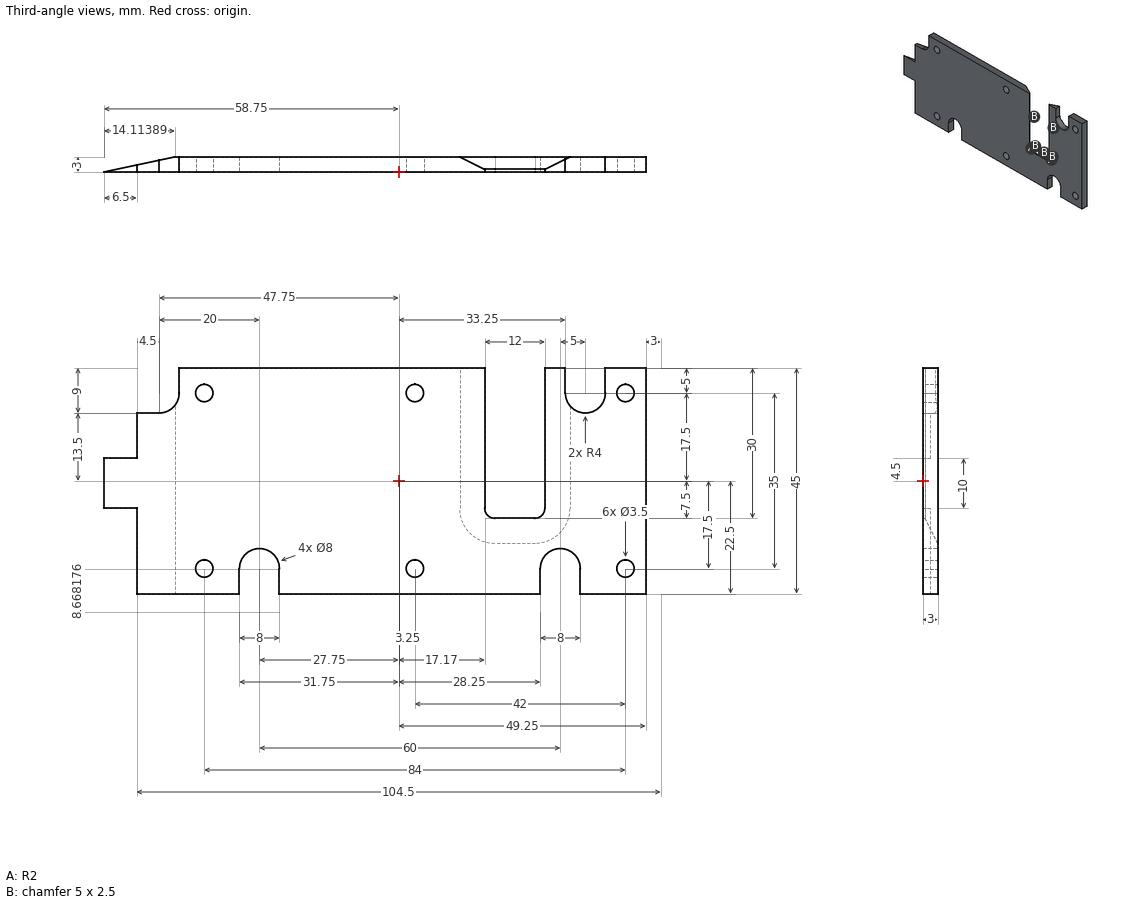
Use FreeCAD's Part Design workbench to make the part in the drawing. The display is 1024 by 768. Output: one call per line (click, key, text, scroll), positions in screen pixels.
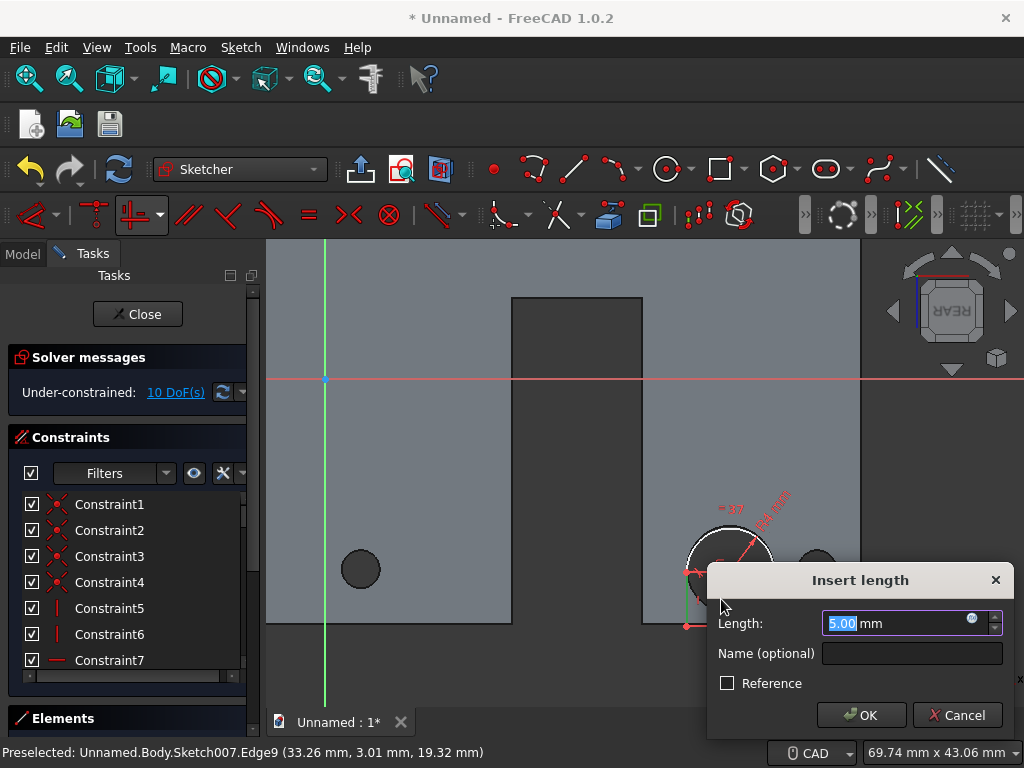
text(5)
key(Return)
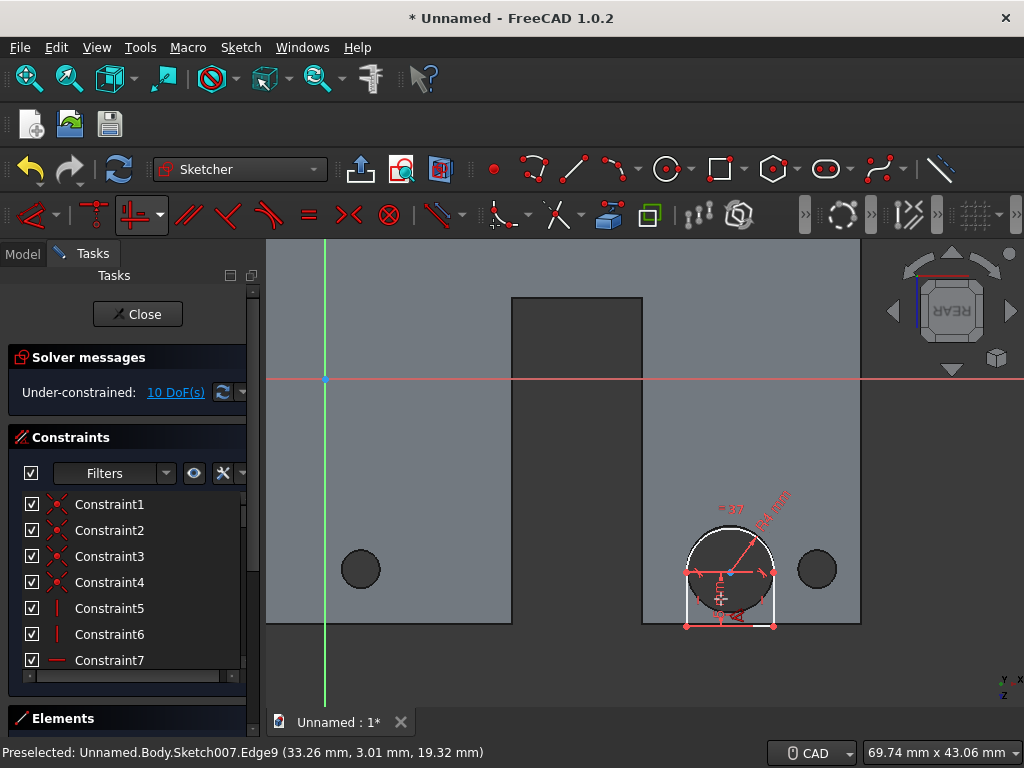
scroll(757, 539, down, 5)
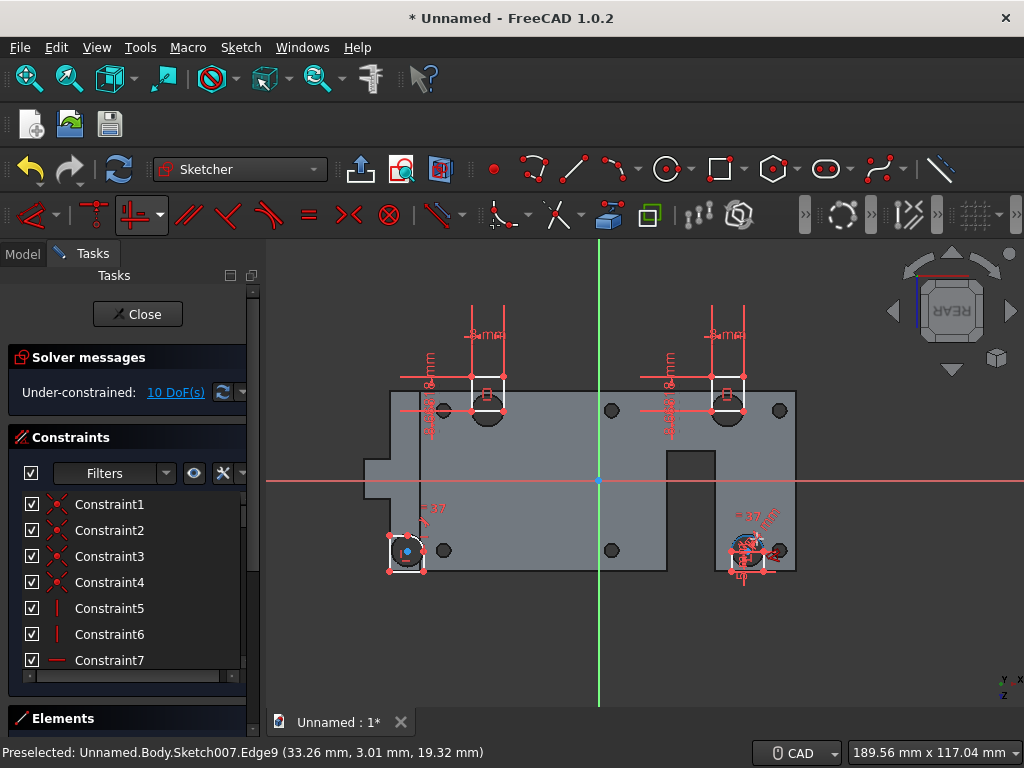
scroll(390, 547, up, 2)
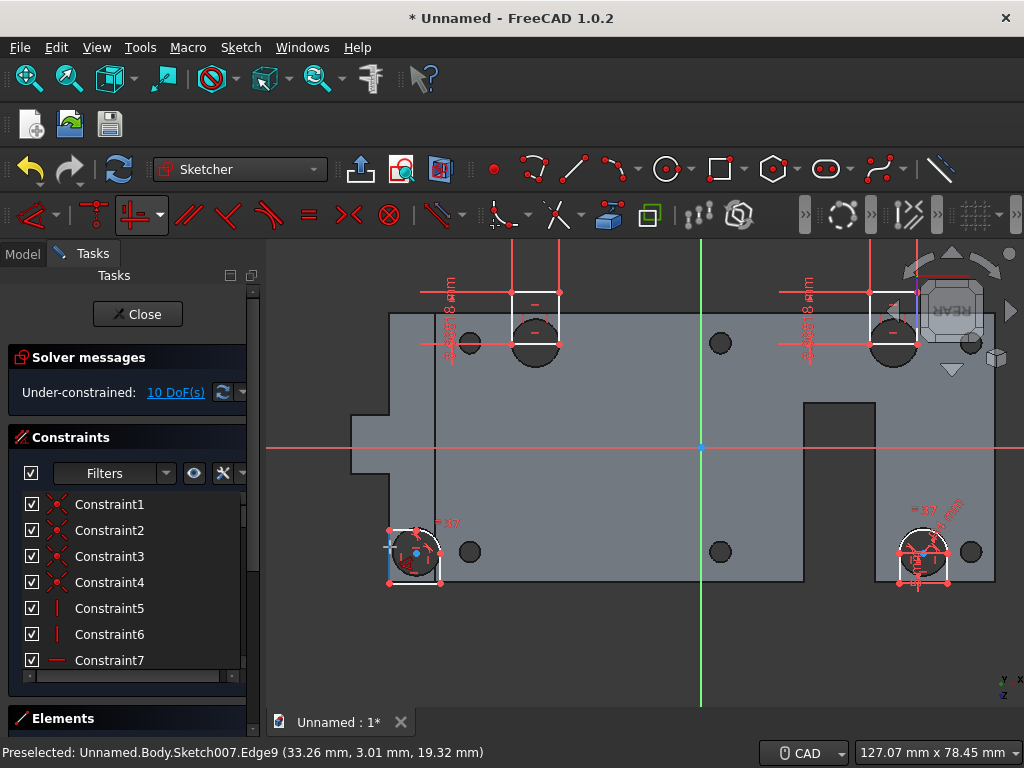
click(389, 546)
click(355, 557)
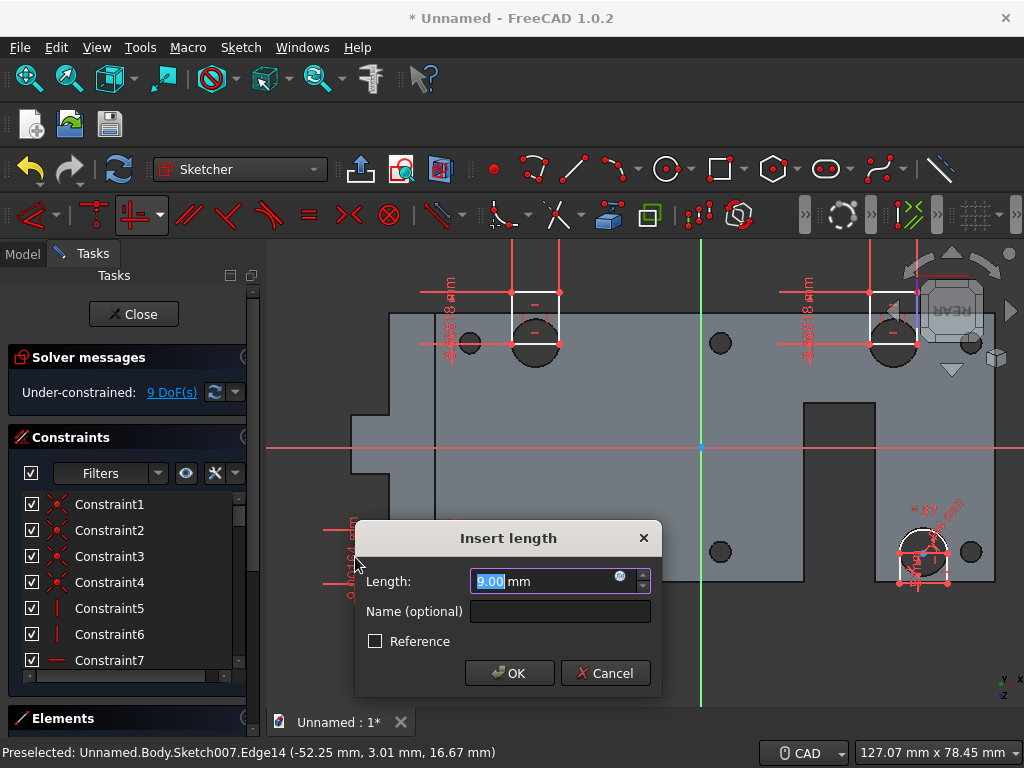
text(9)
key(Return)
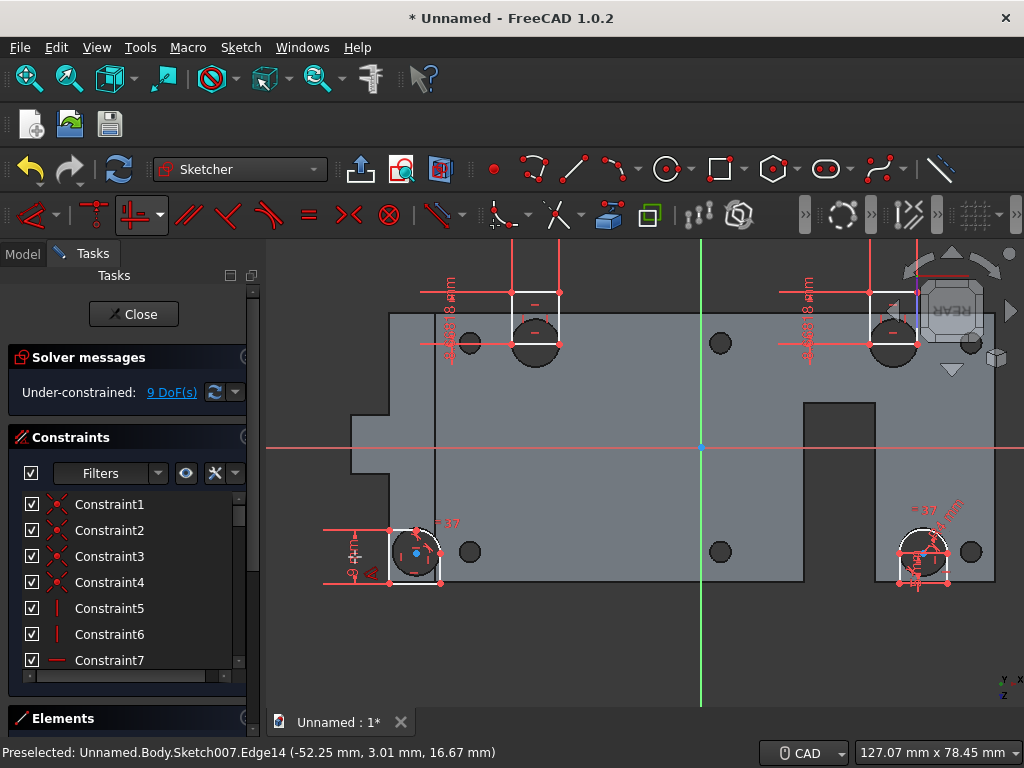
scroll(406, 530, up, 2)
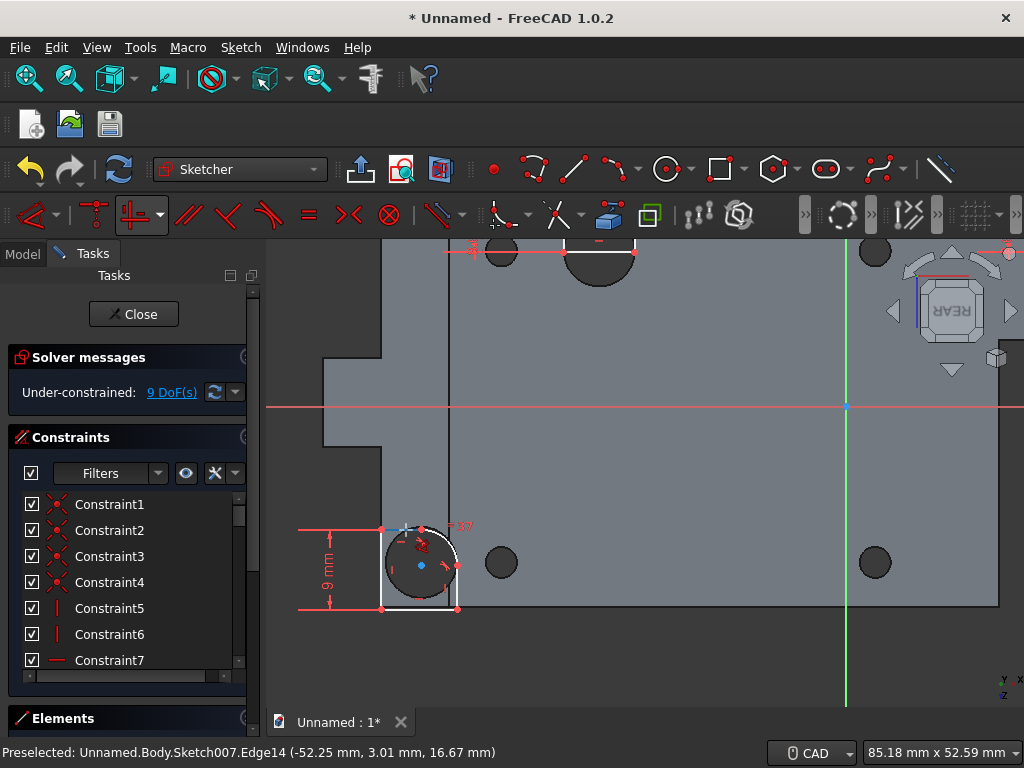
click(405, 530)
click(401, 564)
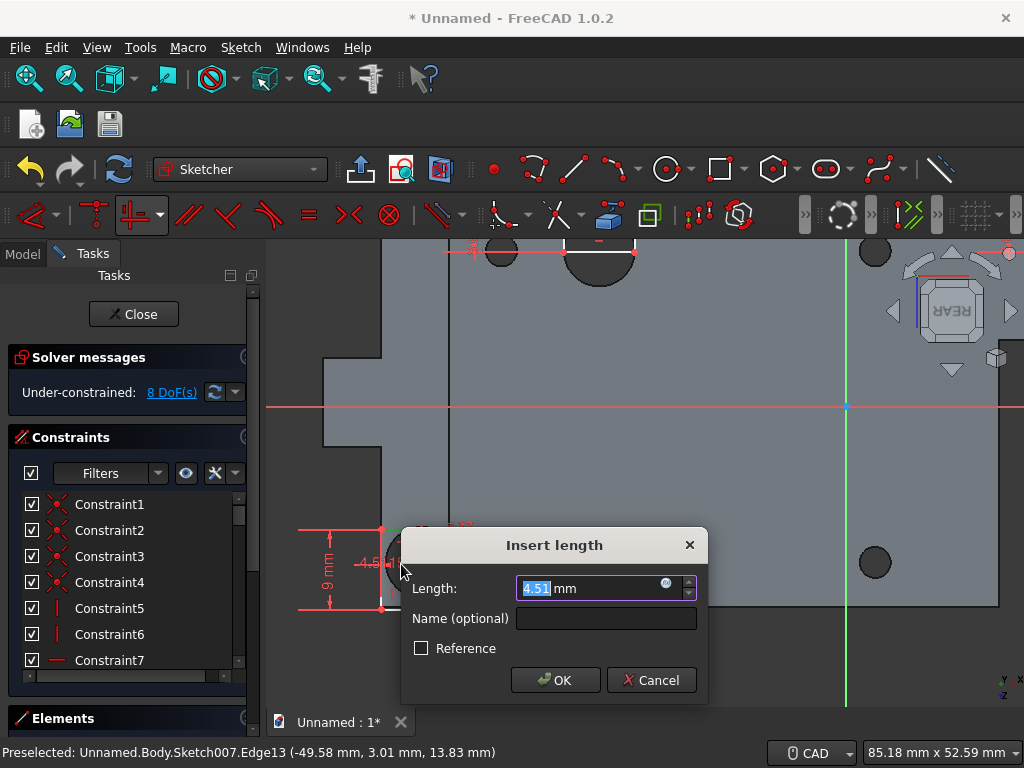
text(4.5)
key(Return)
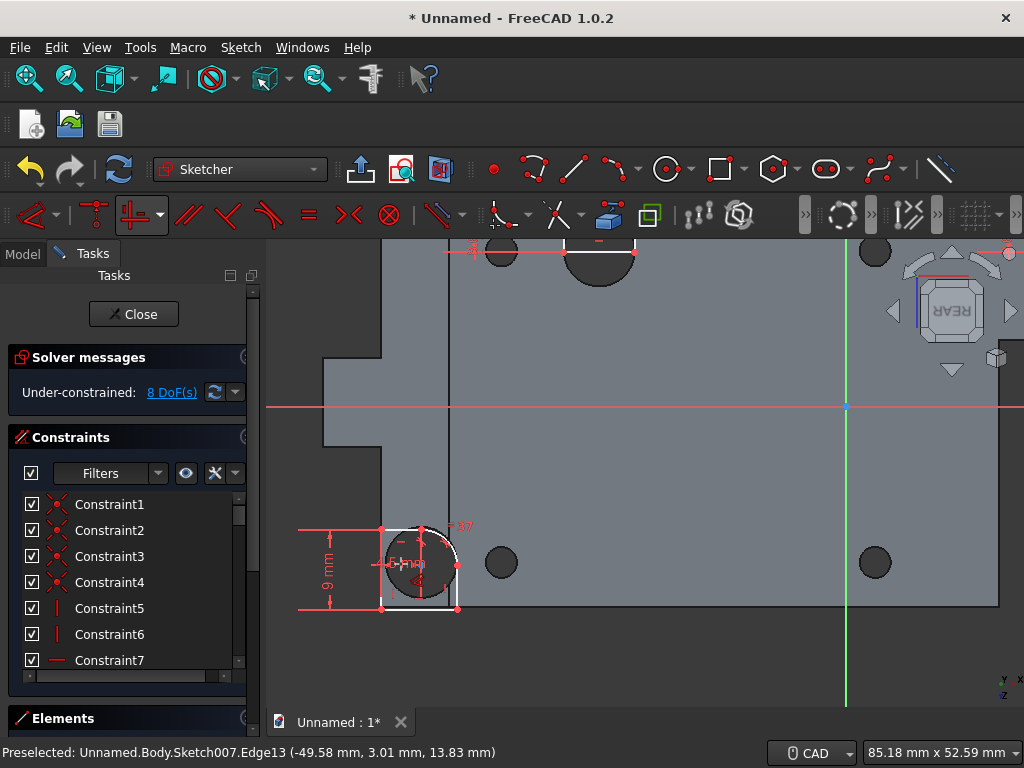
scroll(396, 540, down, 4)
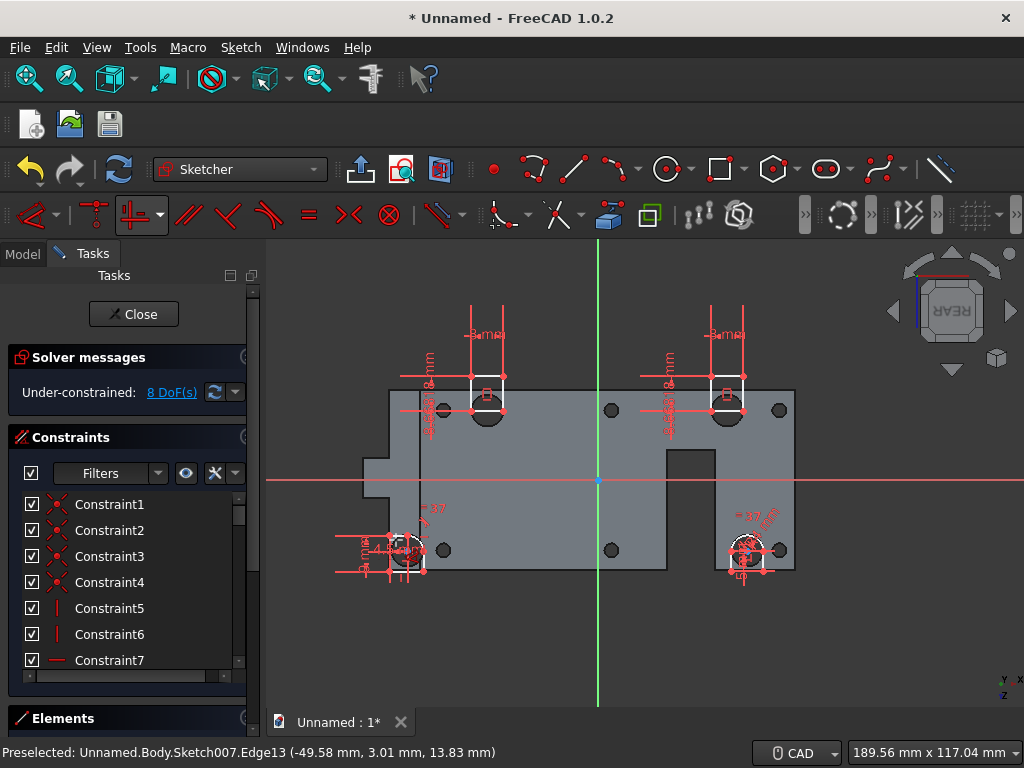
click(471, 411)
click(437, 446)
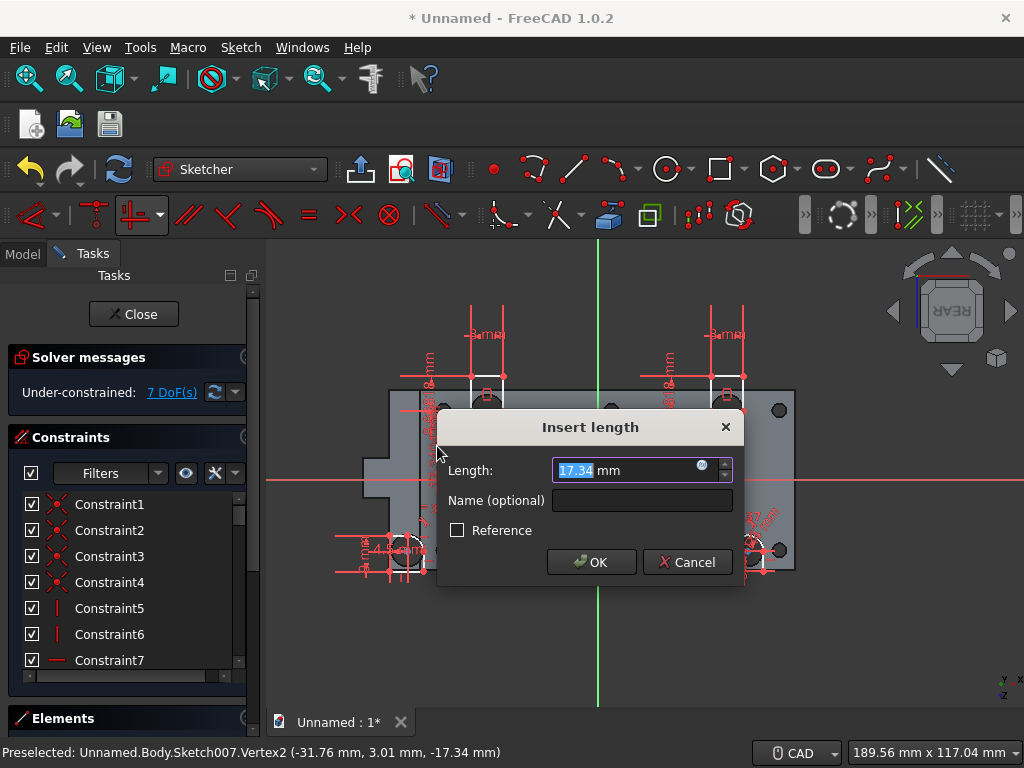
text(17.5)
key(Return)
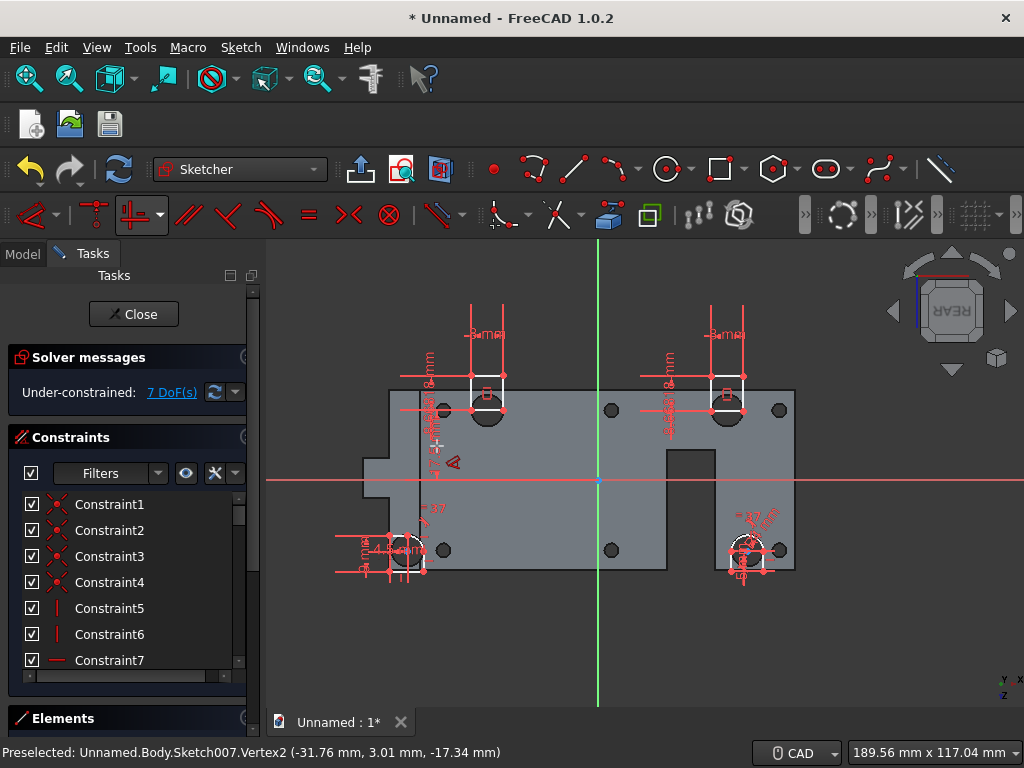
click(711, 411)
click(745, 446)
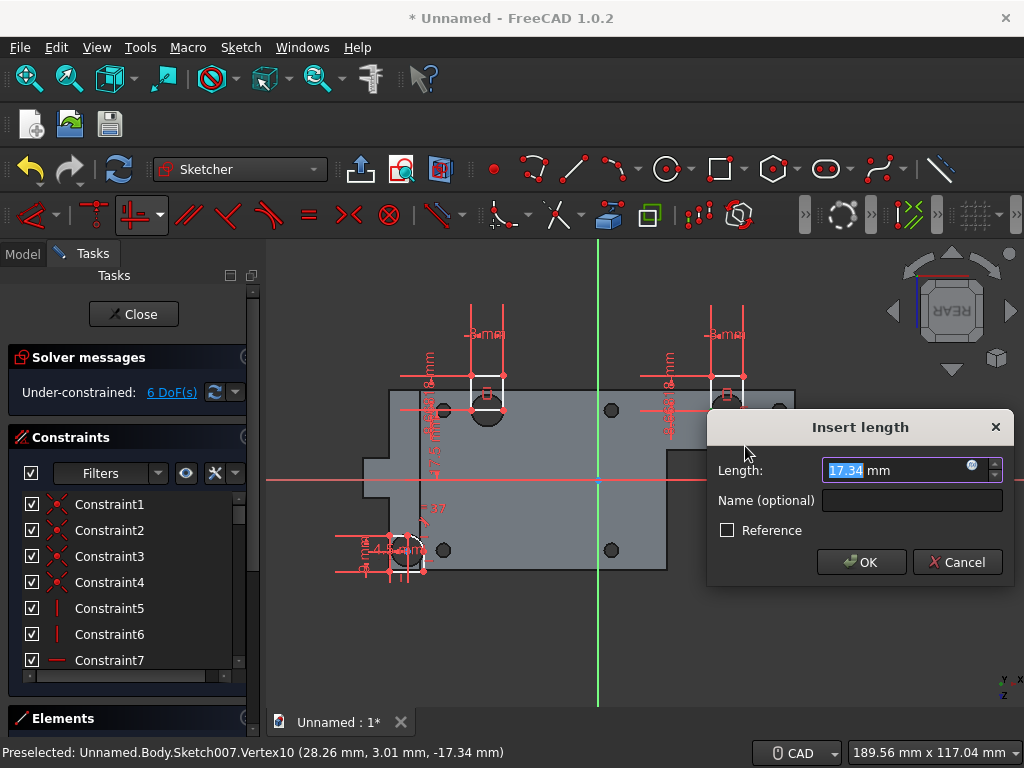
text(17.5)
key(Return)